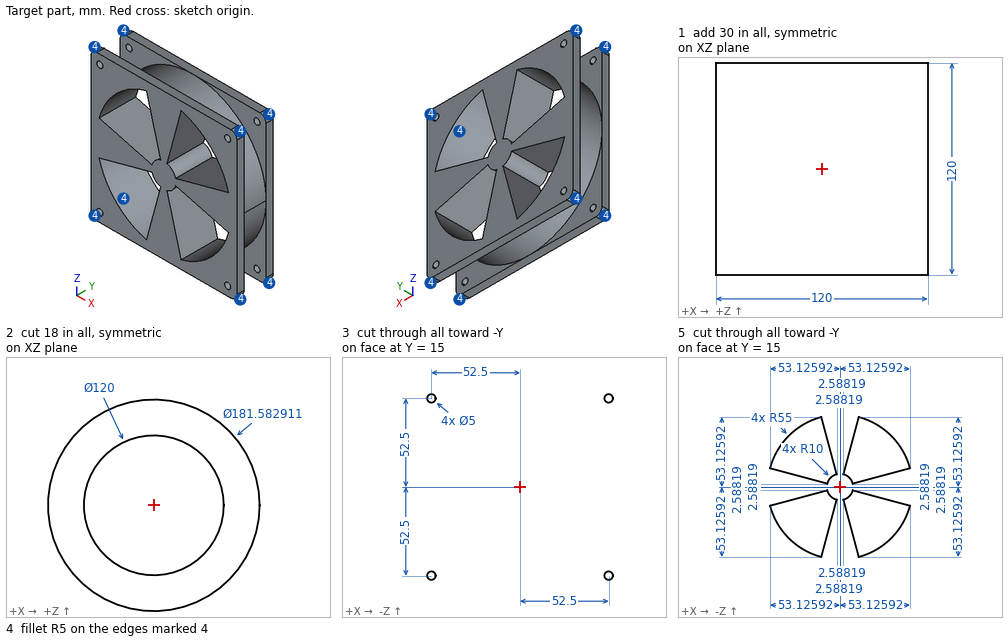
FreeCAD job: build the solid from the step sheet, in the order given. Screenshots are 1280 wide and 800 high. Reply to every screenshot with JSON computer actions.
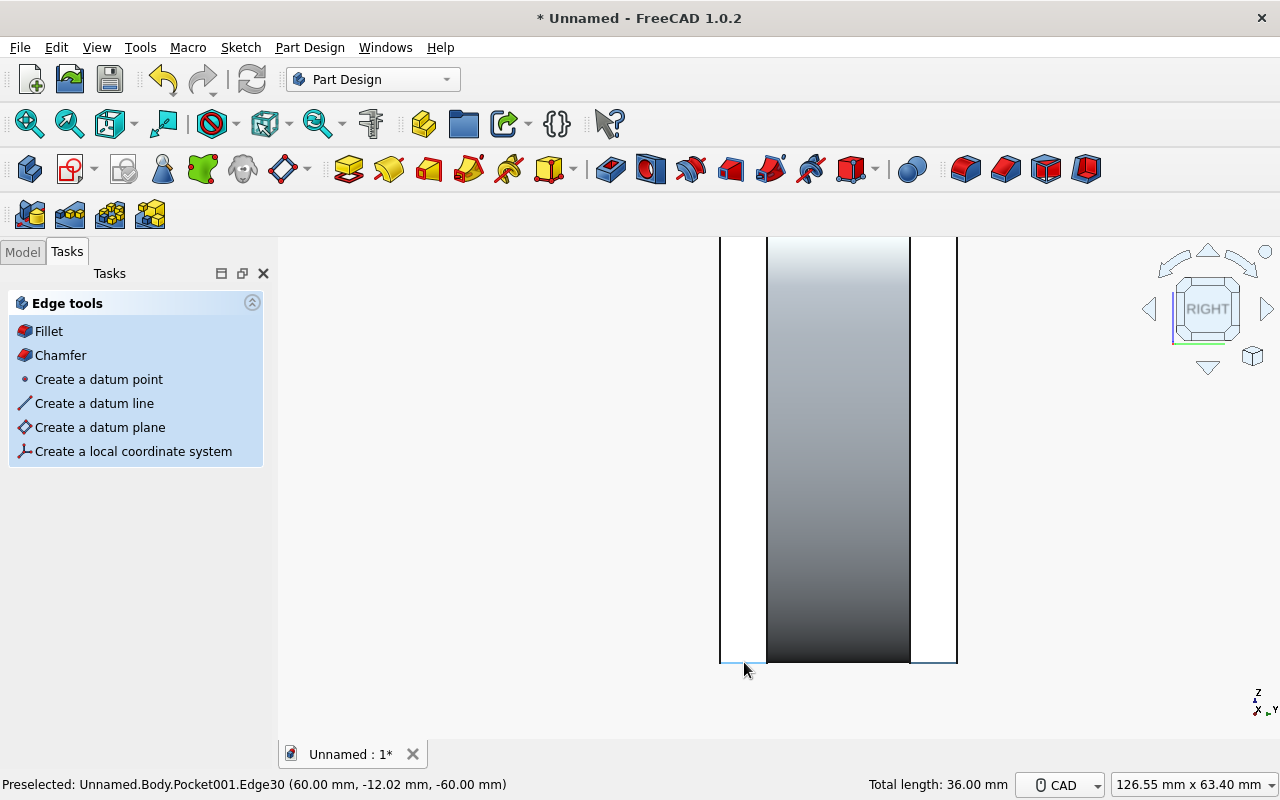
{"action": "left_click", "coordinate": [30, 124]}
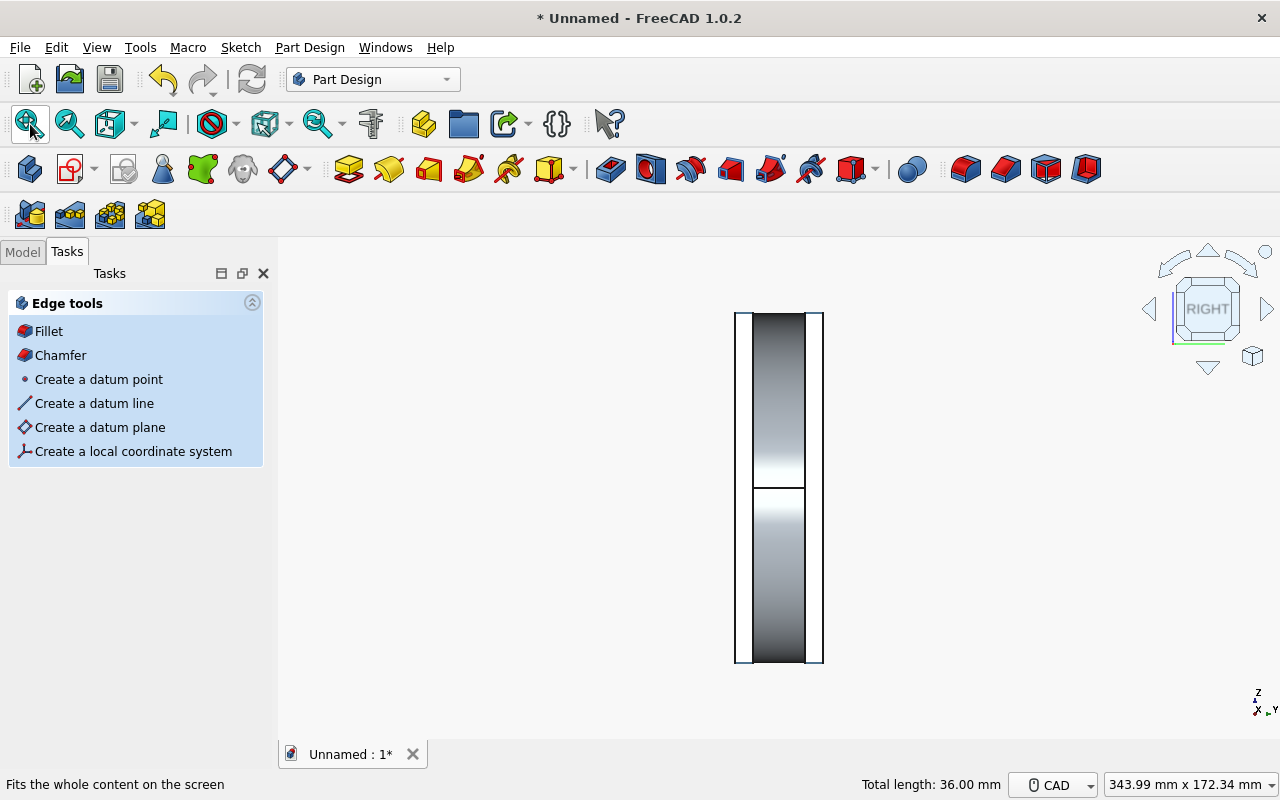
{"action": "key", "text": "5"}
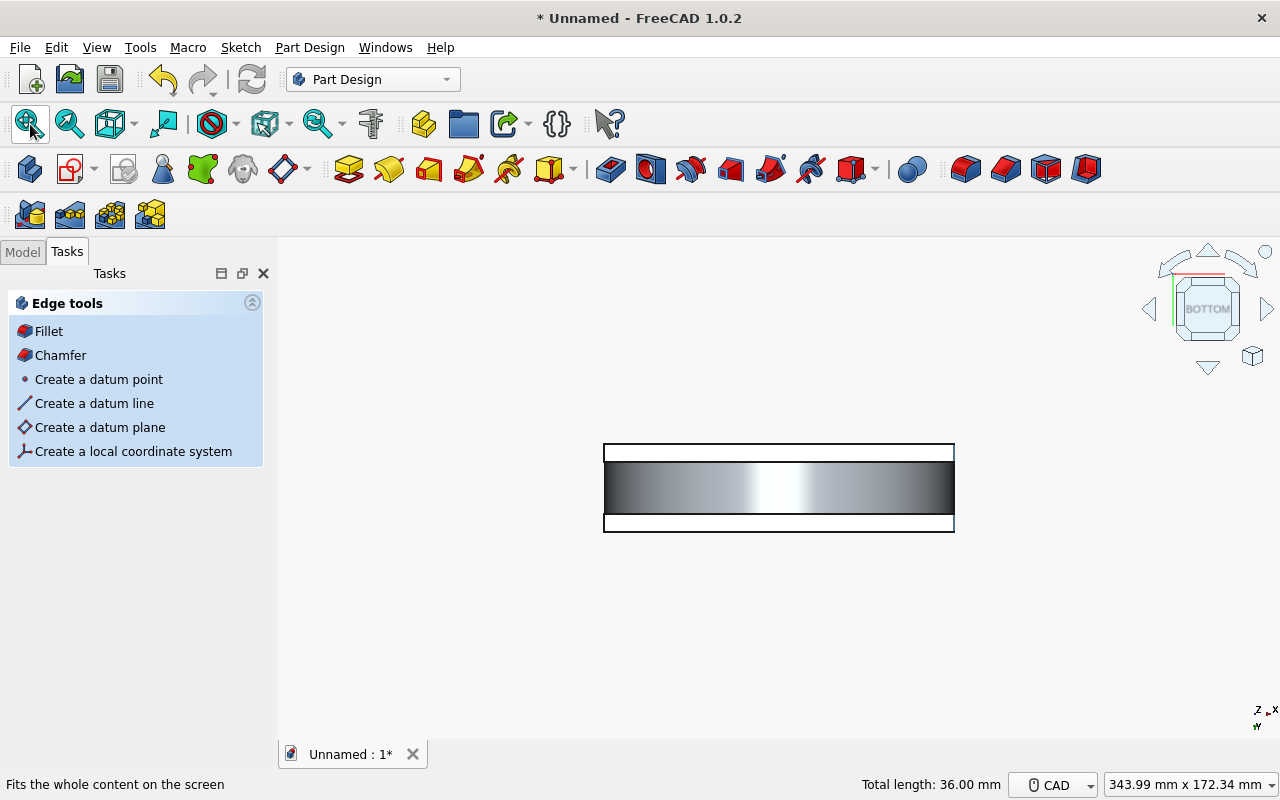
{"action": "left_click", "coordinate": [30, 124]}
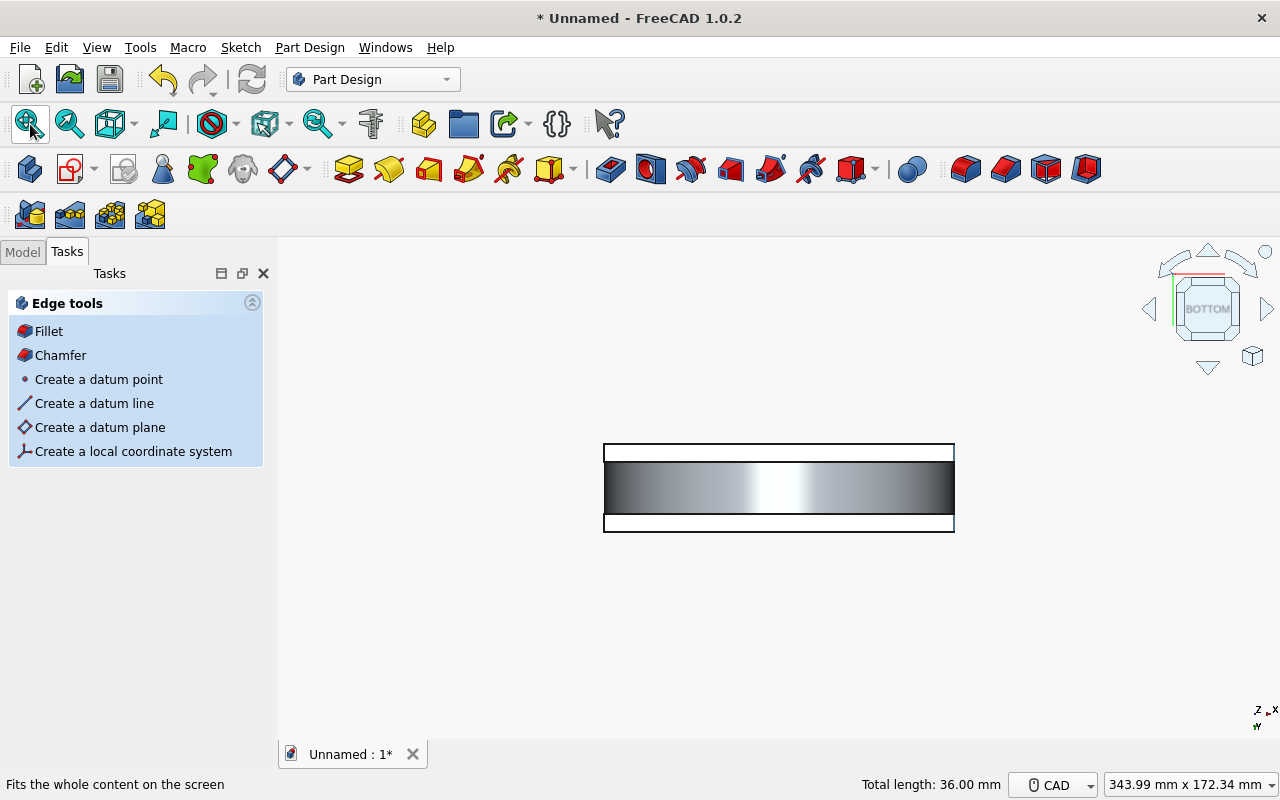
{"action": "left_click", "coordinate": [604, 452], "text": "ctrl"}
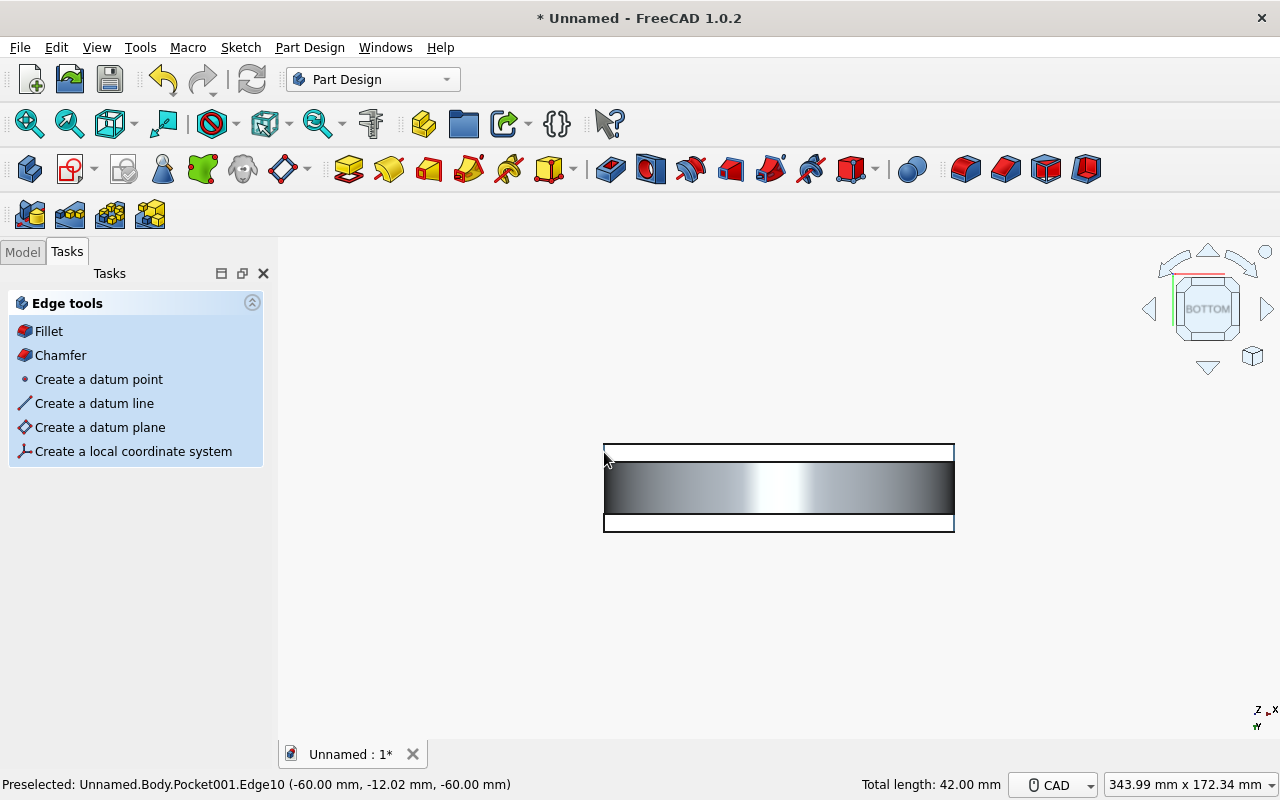
{"action": "left_click", "coordinate": [604, 522], "text": "ctrl"}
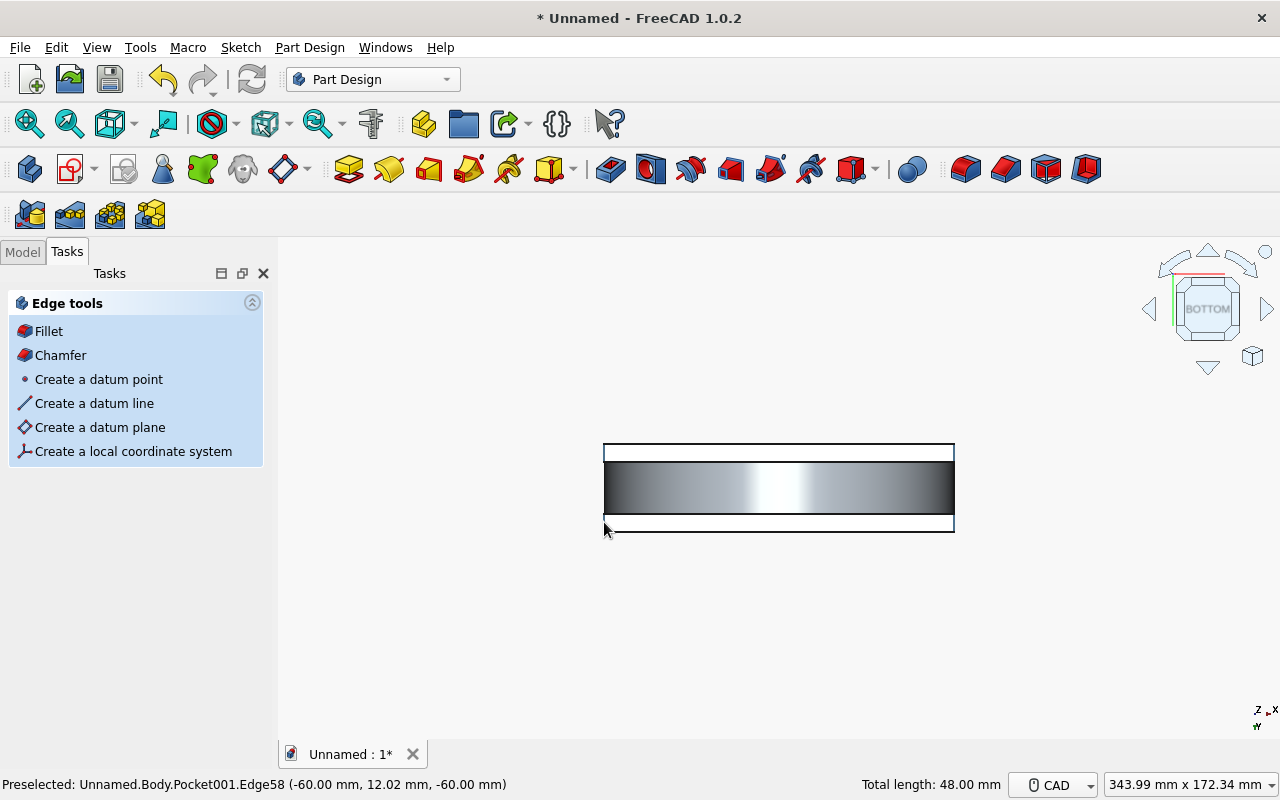
{"action": "left_click", "coordinate": [966, 170]}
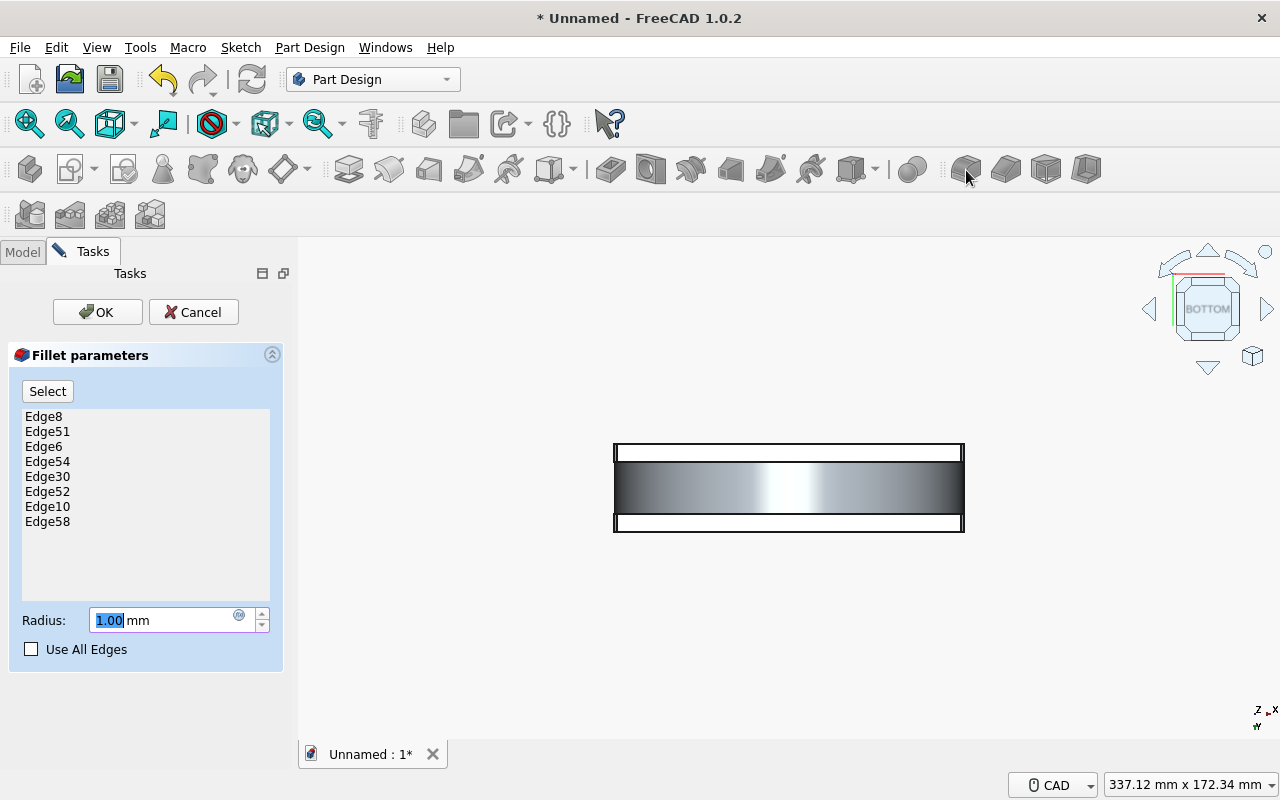
{"action": "type", "text": "5"}
{"action": "key", "text": "Tab"}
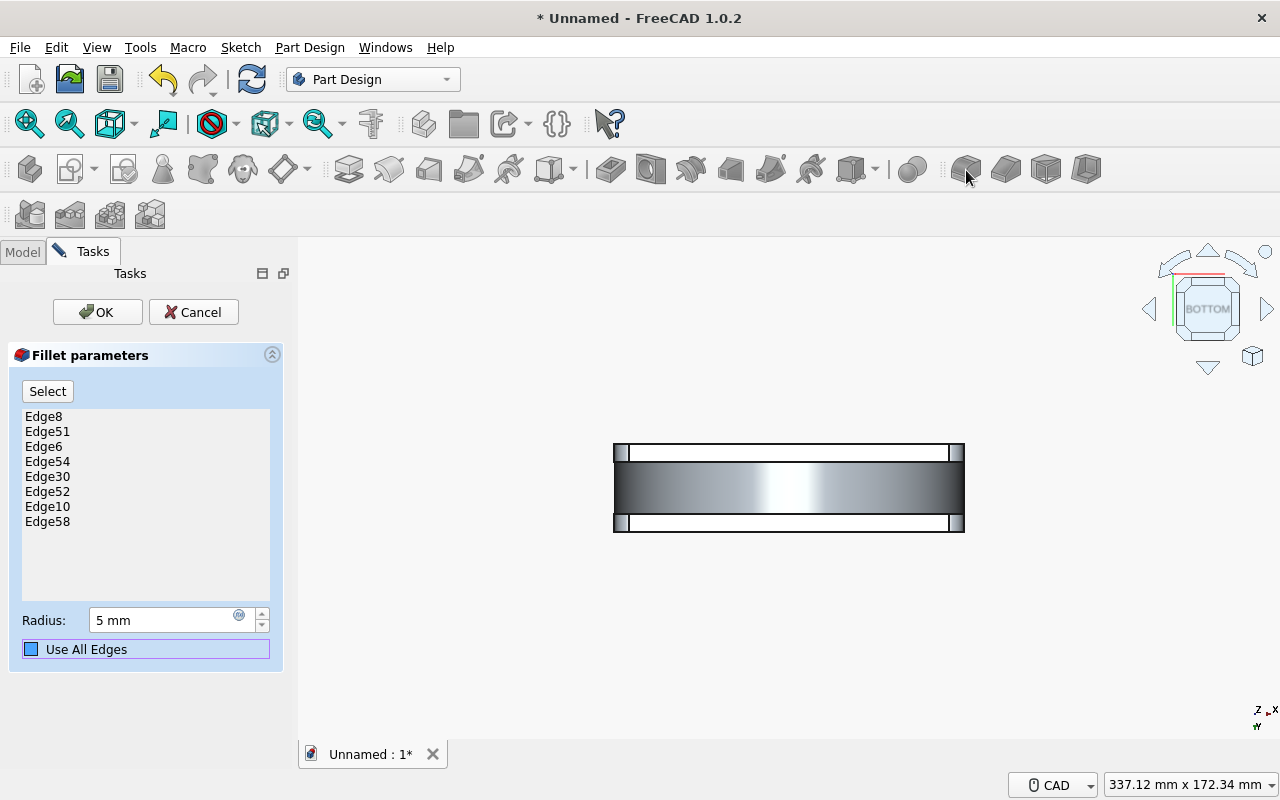
{"action": "left_click", "coordinate": [98, 312]}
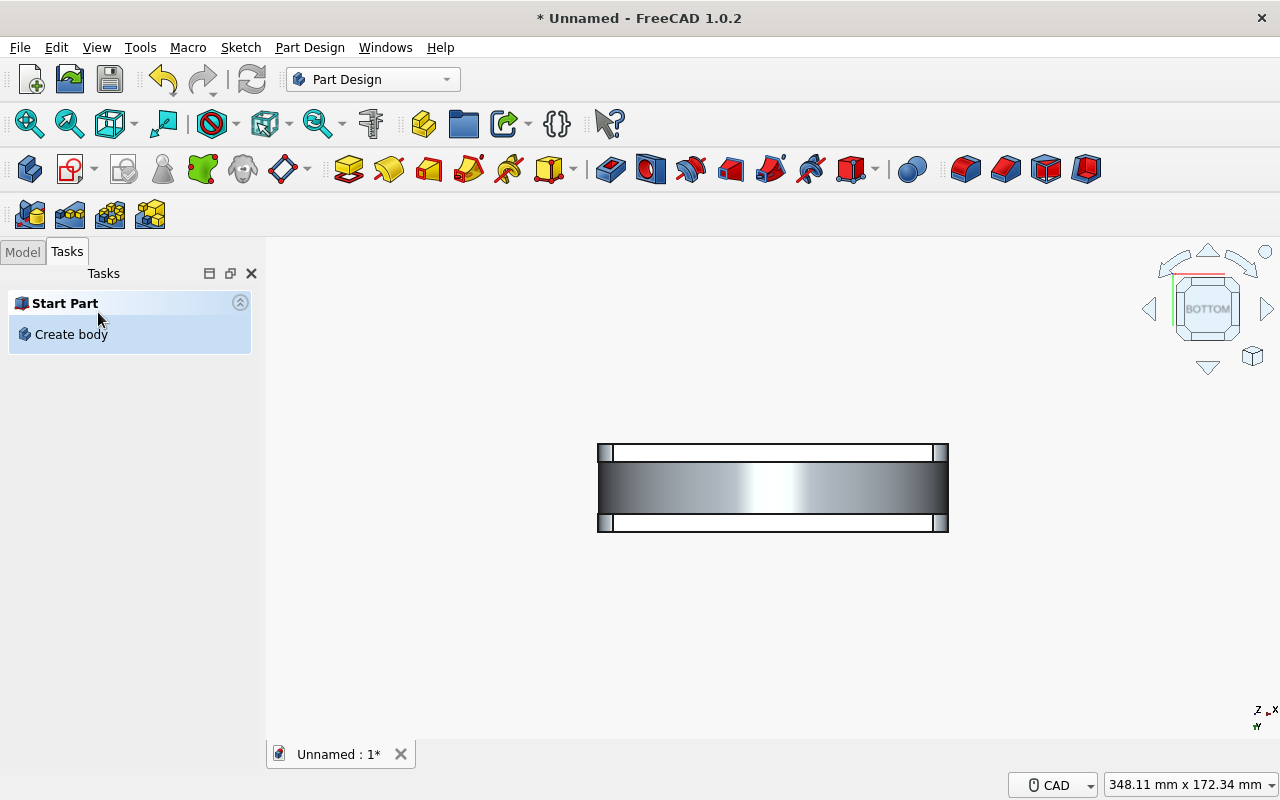
{"action": "left_click", "coordinate": [30, 124]}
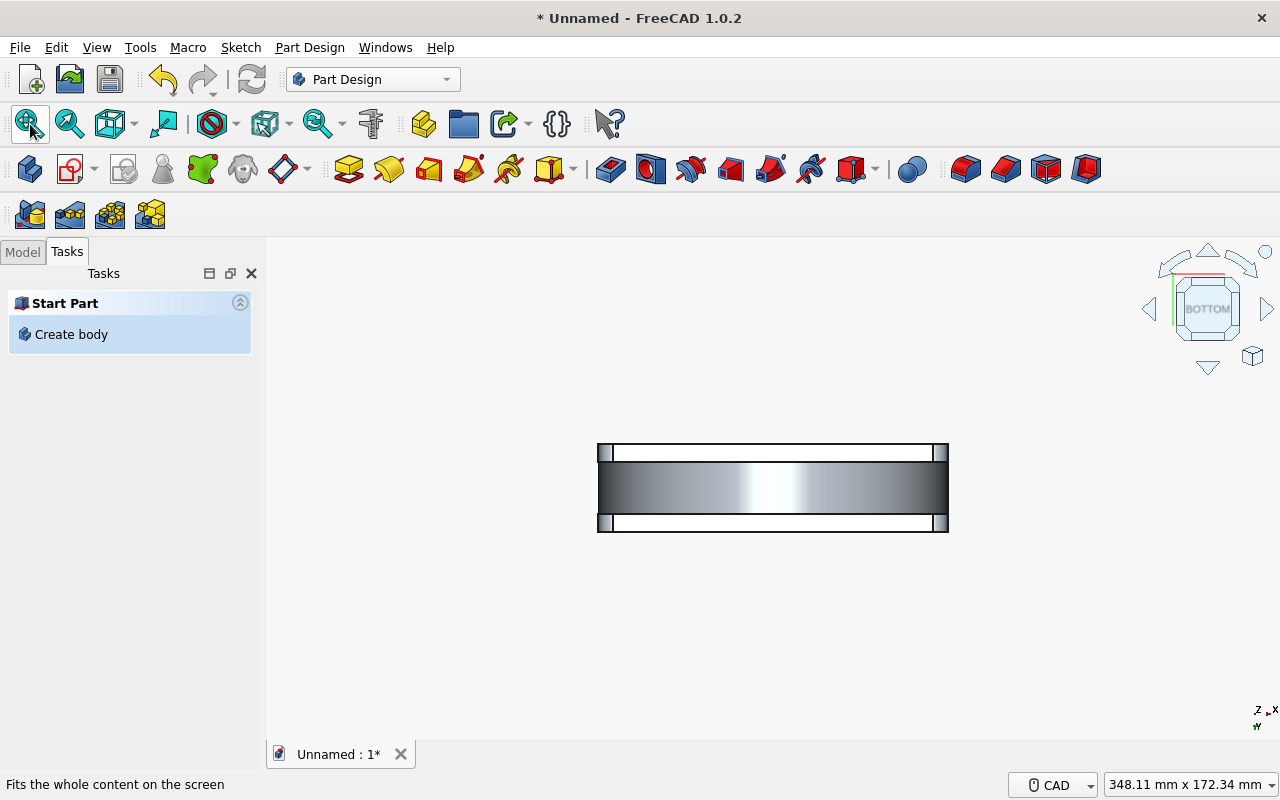
{"action": "key", "text": "4"}